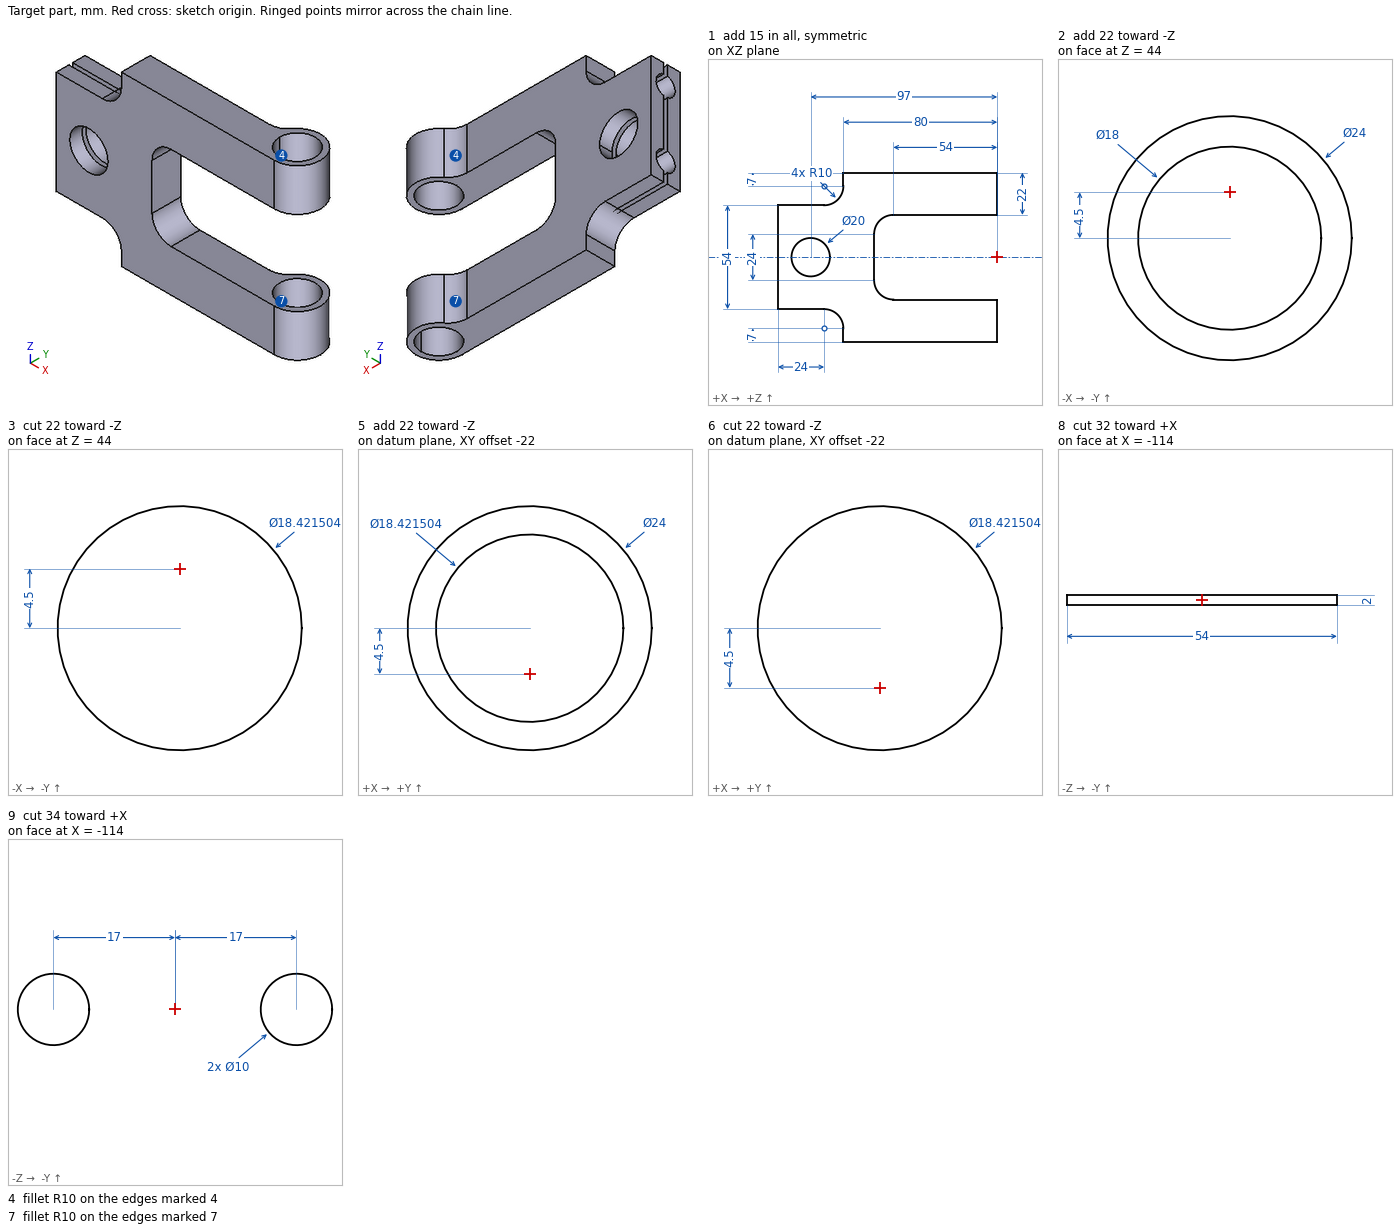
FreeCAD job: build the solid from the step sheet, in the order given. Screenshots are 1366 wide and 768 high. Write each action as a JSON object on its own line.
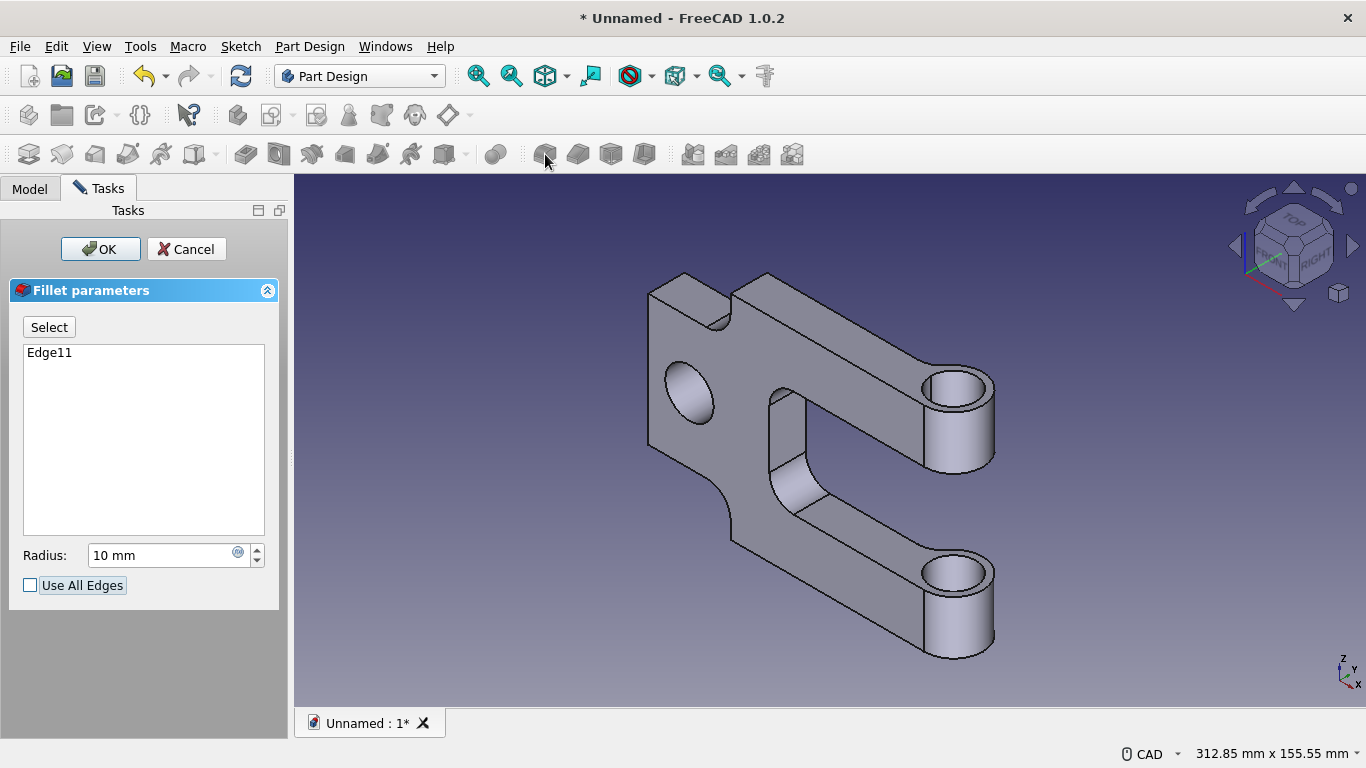
{"action": "left_click", "coordinate": [101, 249]}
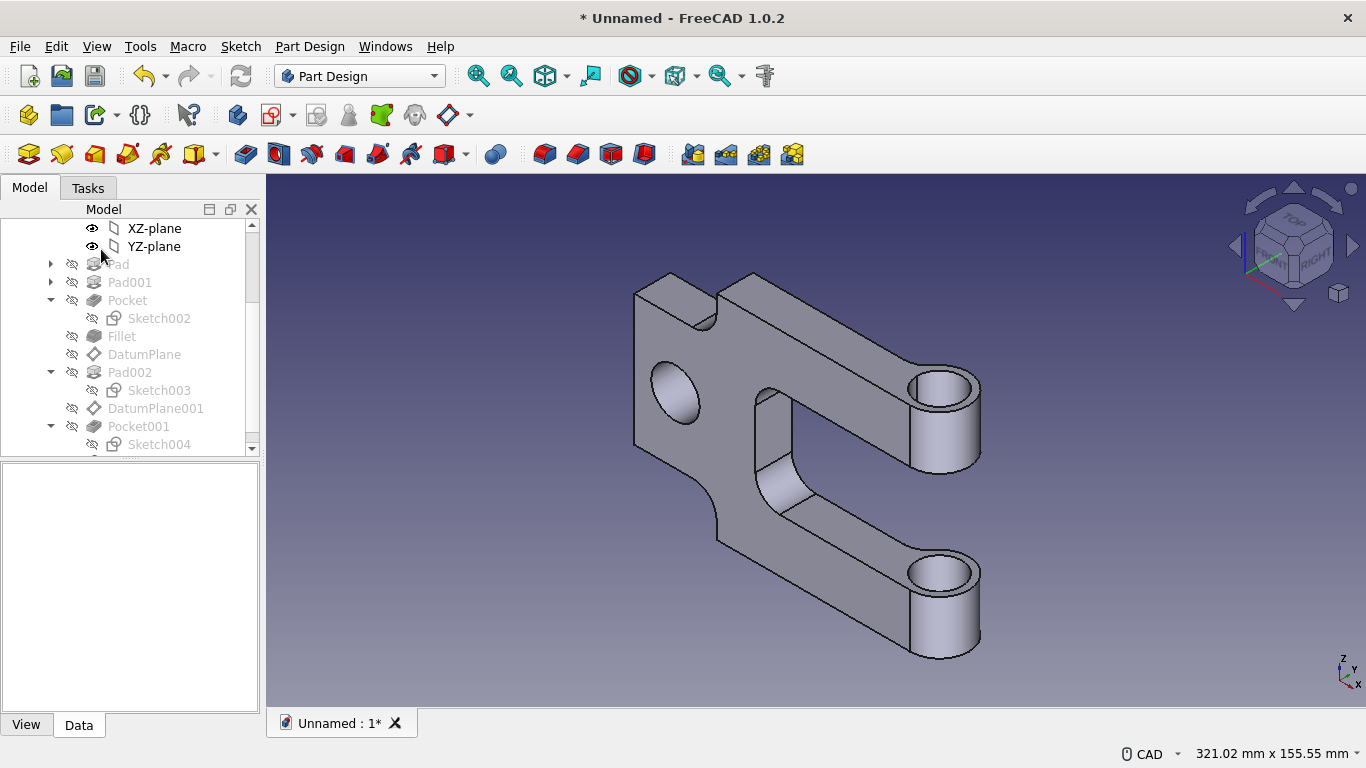
{"action": "key", "text": "6"}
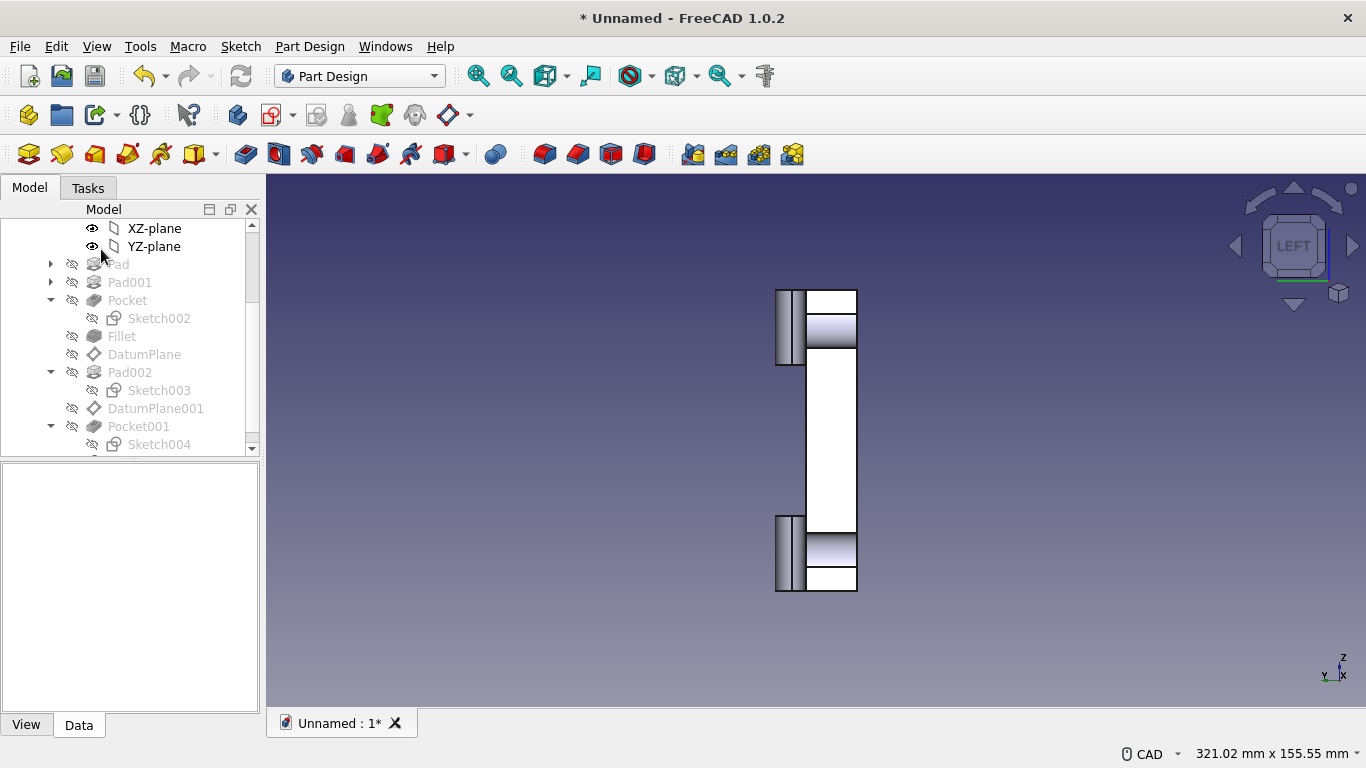
{"action": "left_click", "coordinate": [831, 439]}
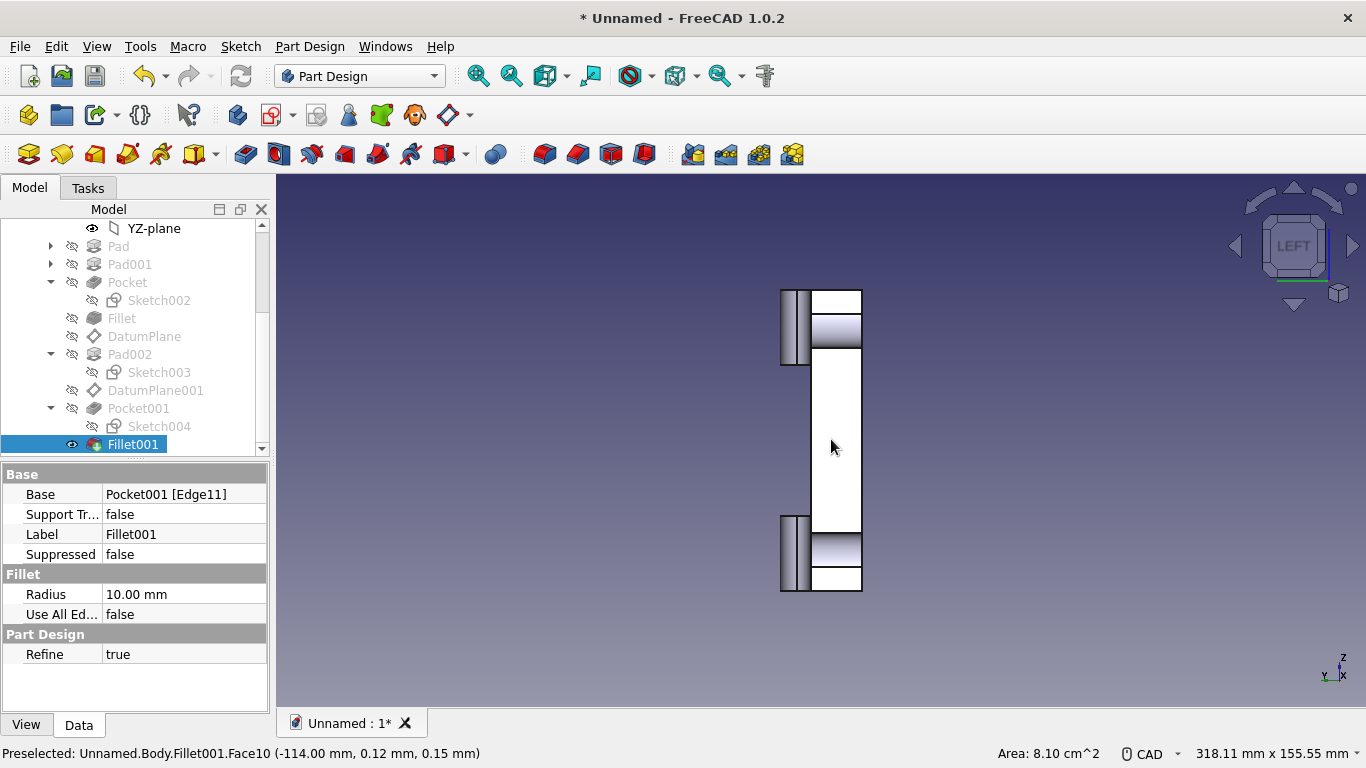
{"action": "left_click", "coordinate": [270, 116]}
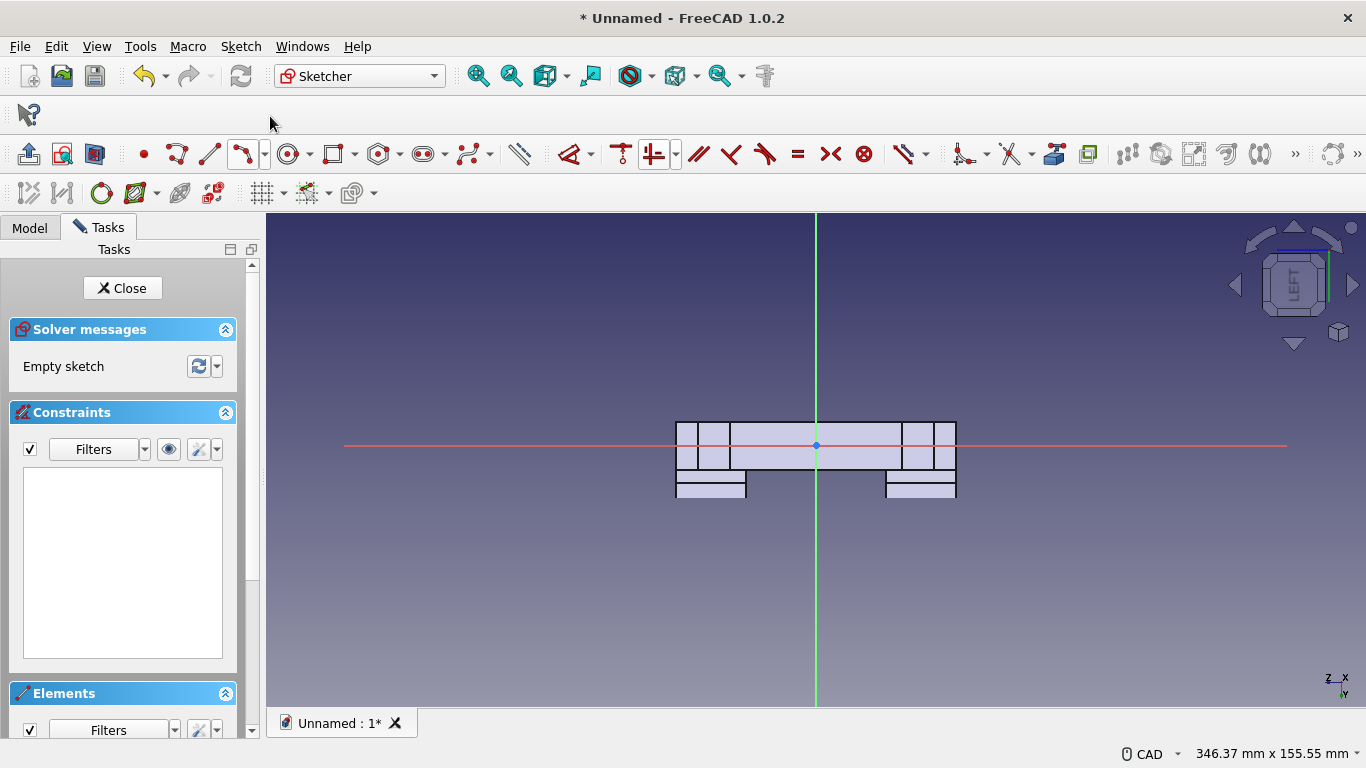
{"action": "scroll", "coordinate": [838, 441], "scroll_direction": "up", "scroll_amount": 7}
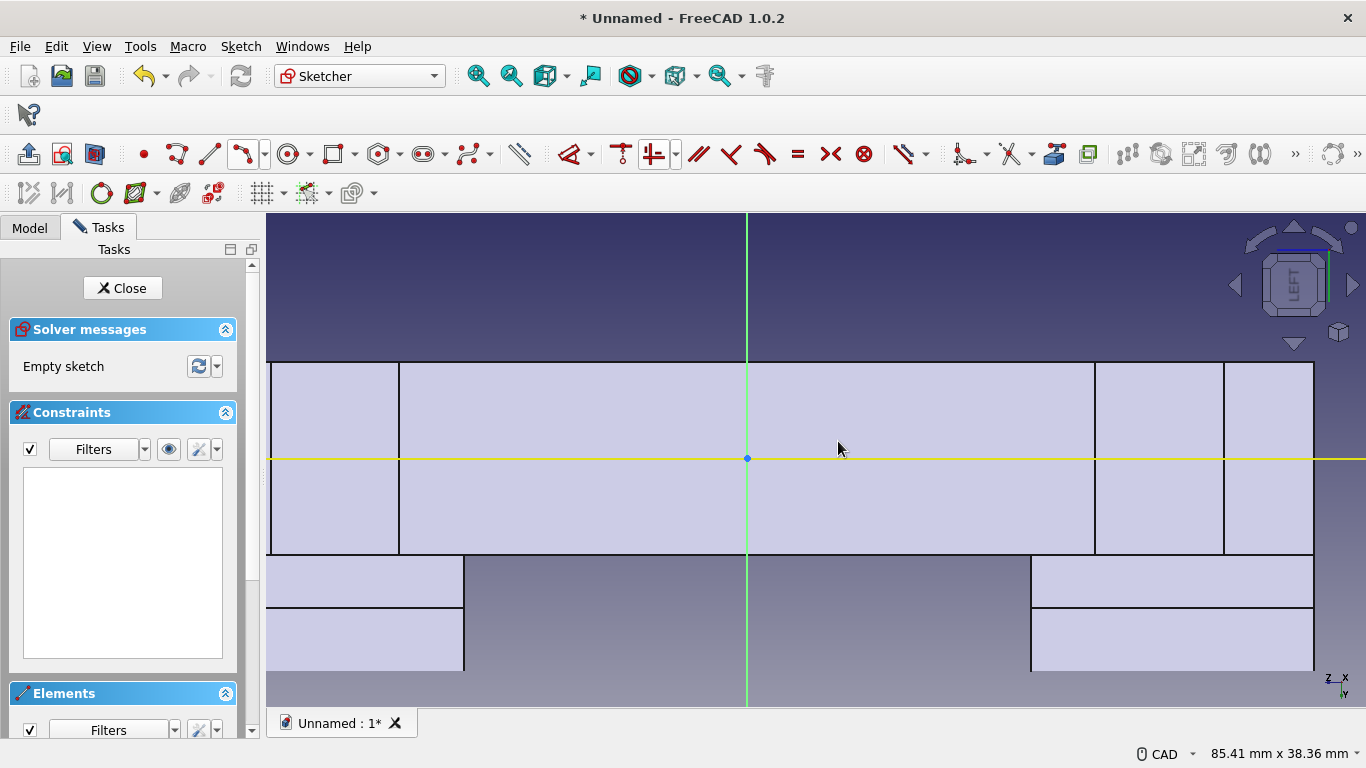
{"action": "key", "text": "g v"}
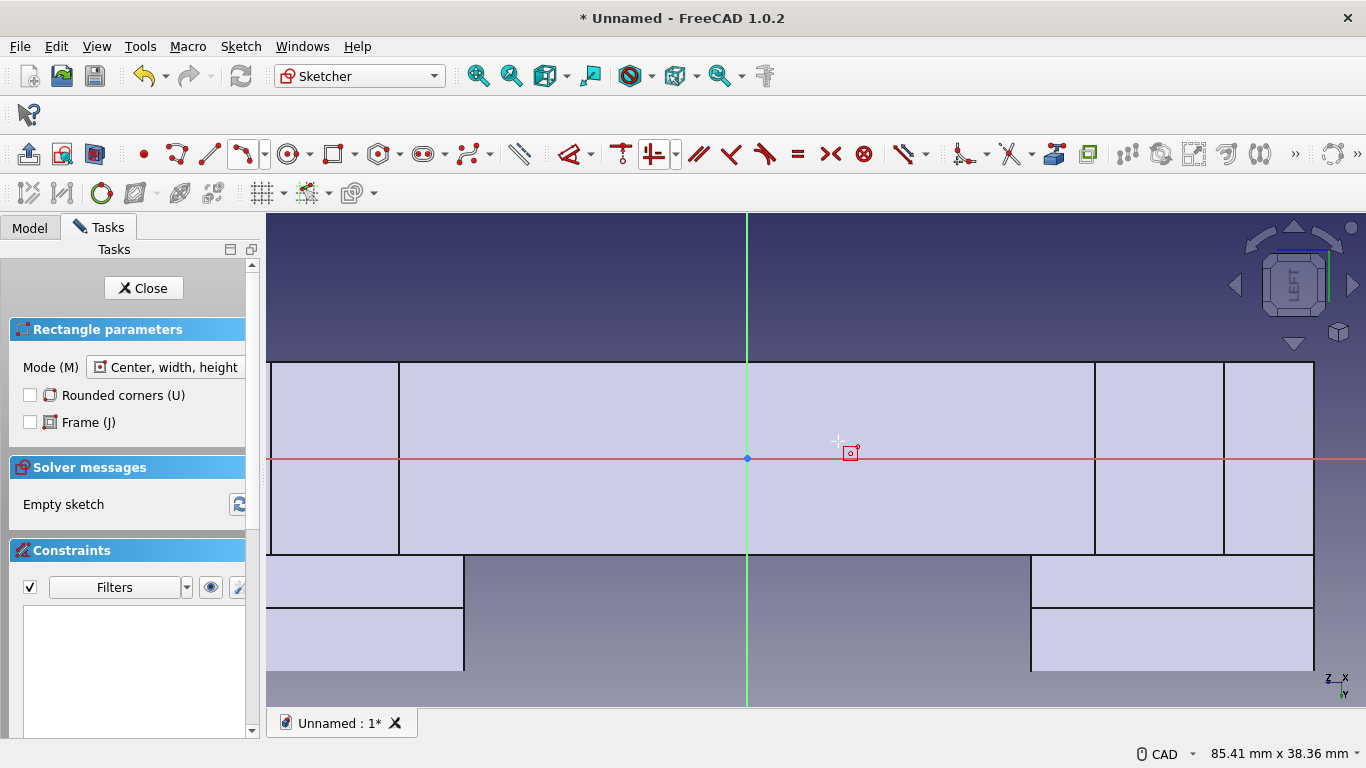
{"action": "scroll", "coordinate": [747, 459], "scroll_direction": "up", "scroll_amount": 2}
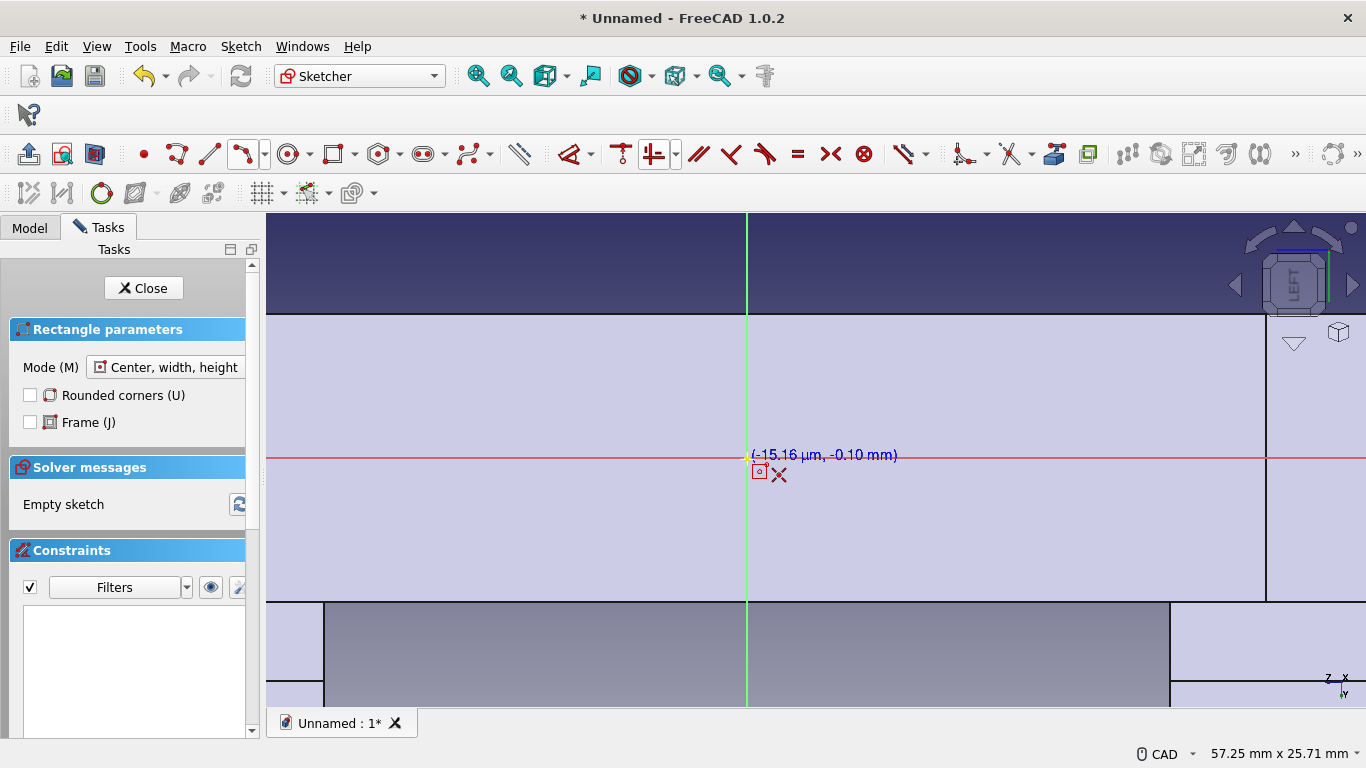
{"action": "left_click", "coordinate": [747, 458]}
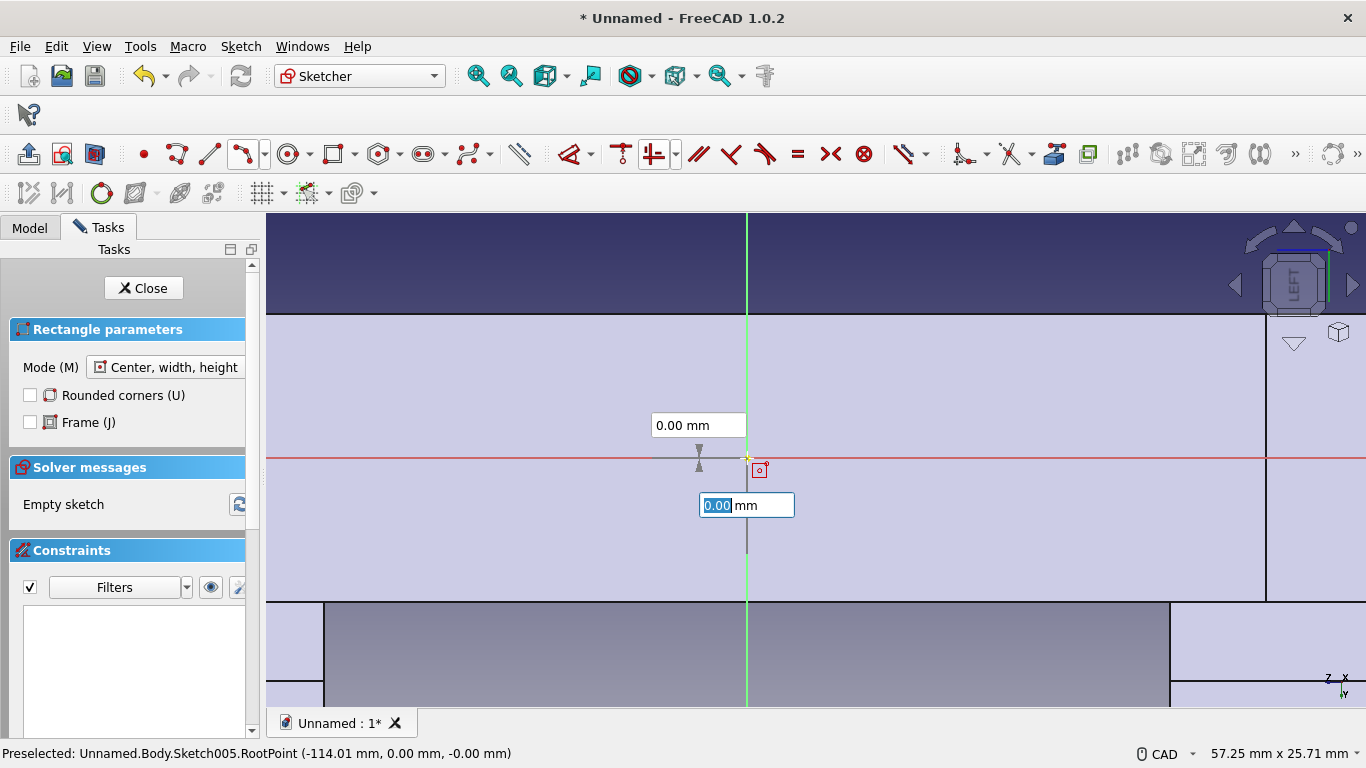
{"action": "scroll", "coordinate": [748, 463], "scroll_direction": "down", "scroll_amount": 2}